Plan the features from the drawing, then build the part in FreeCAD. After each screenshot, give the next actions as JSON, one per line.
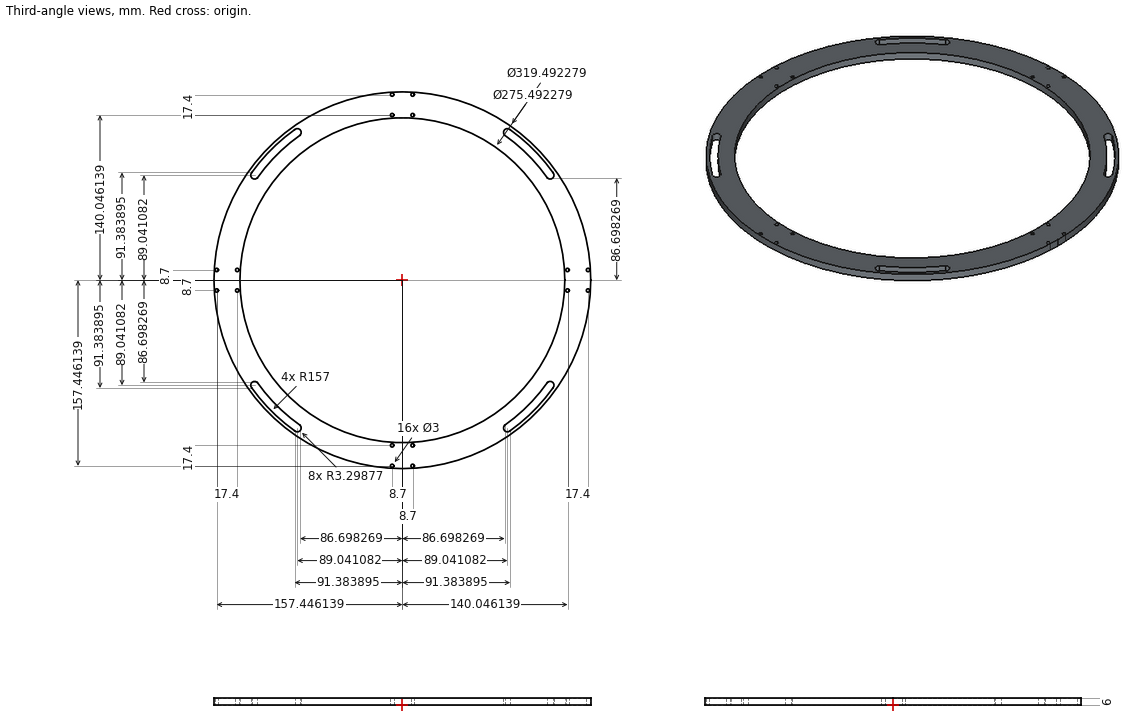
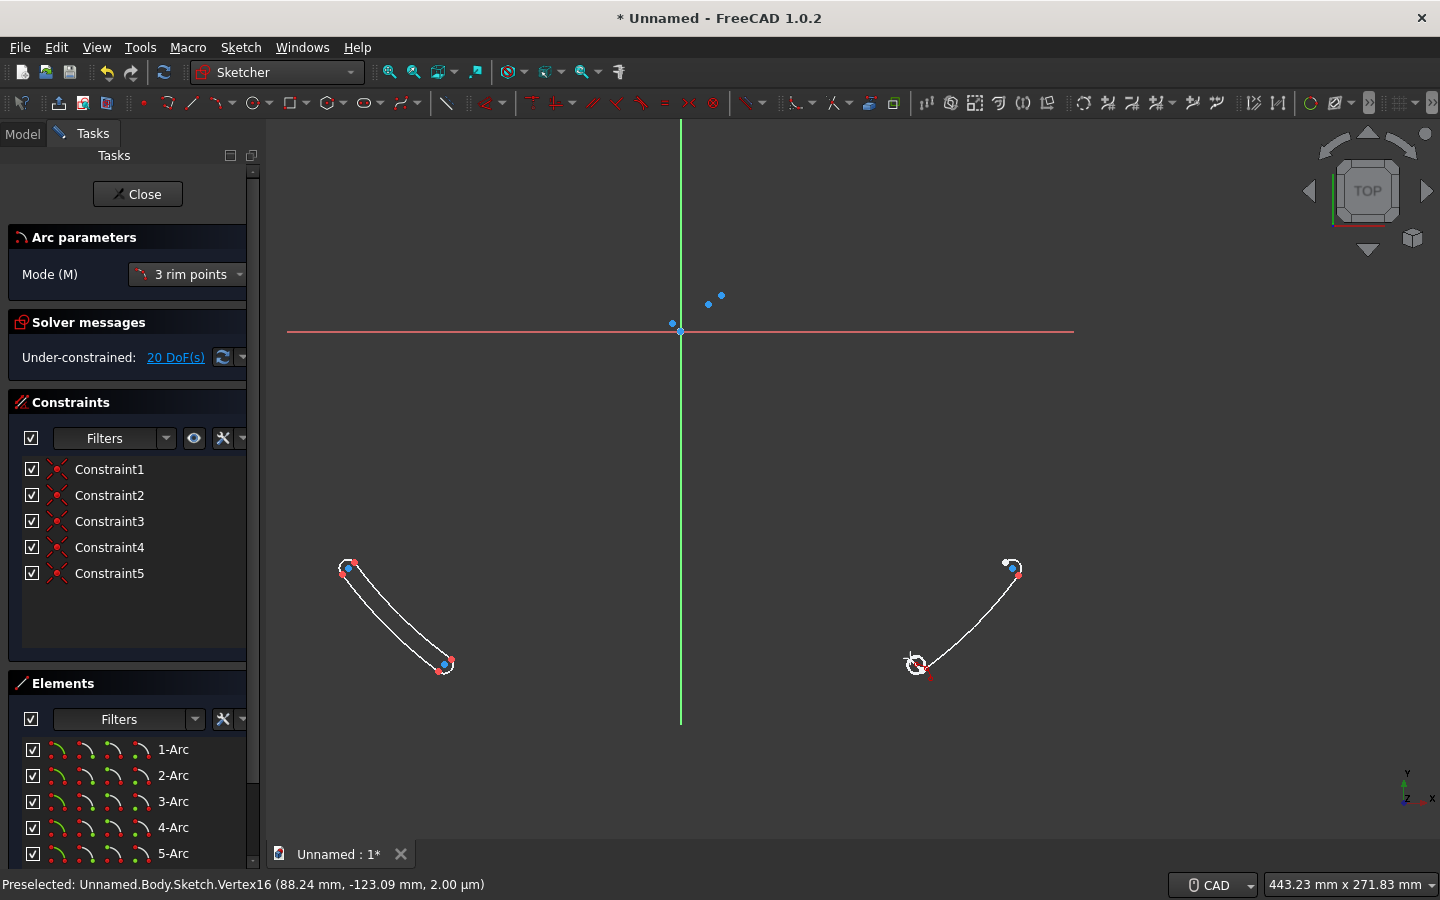
{"action": "scroll", "coordinate": [910, 670], "scroll_direction": "up", "scroll_amount": 3}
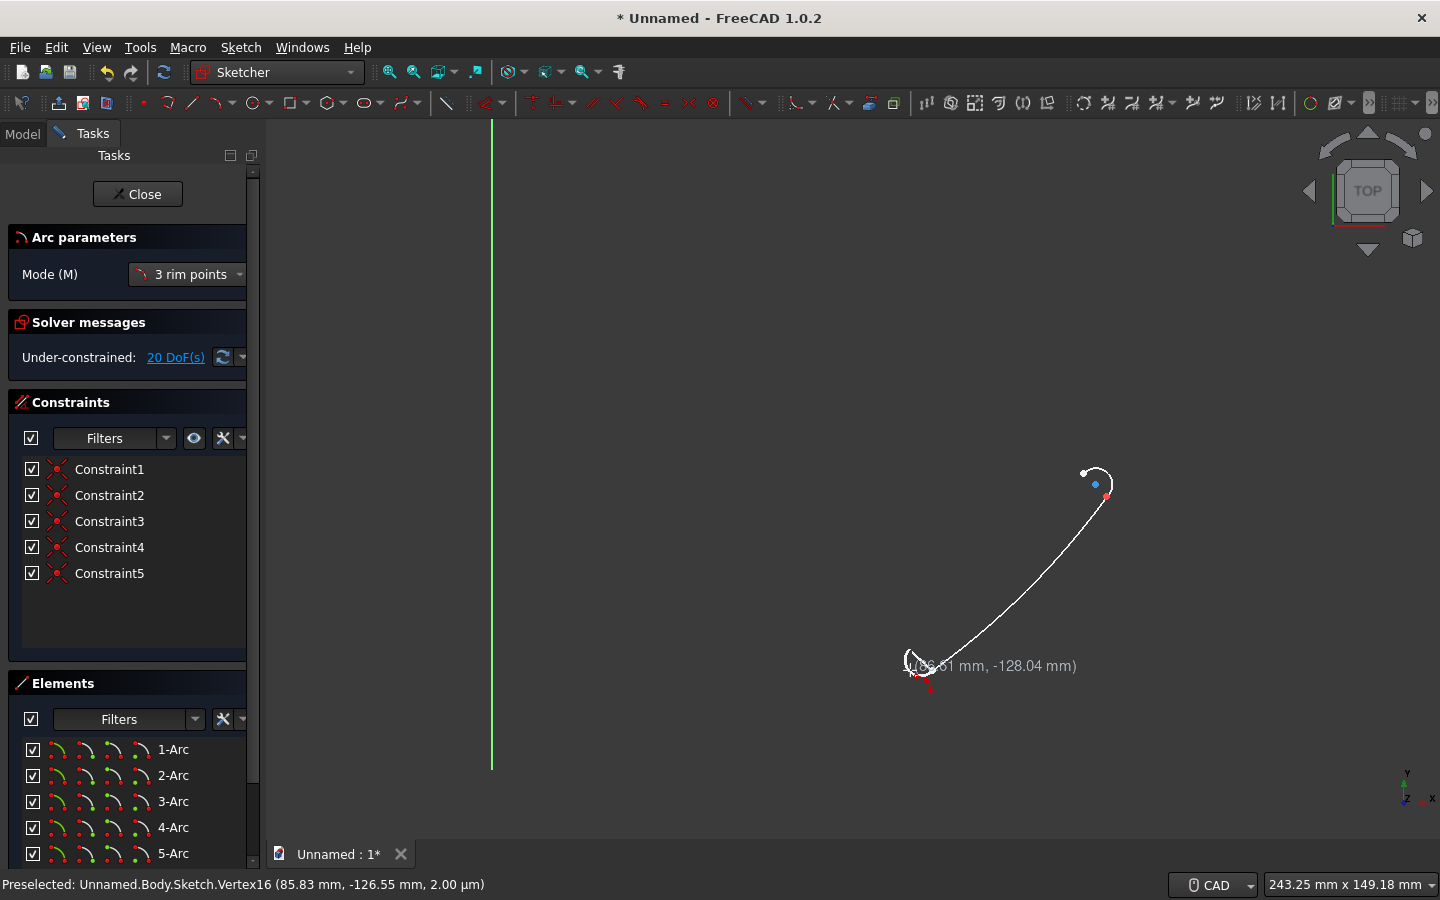
{"action": "left_click", "coordinate": [910, 669]}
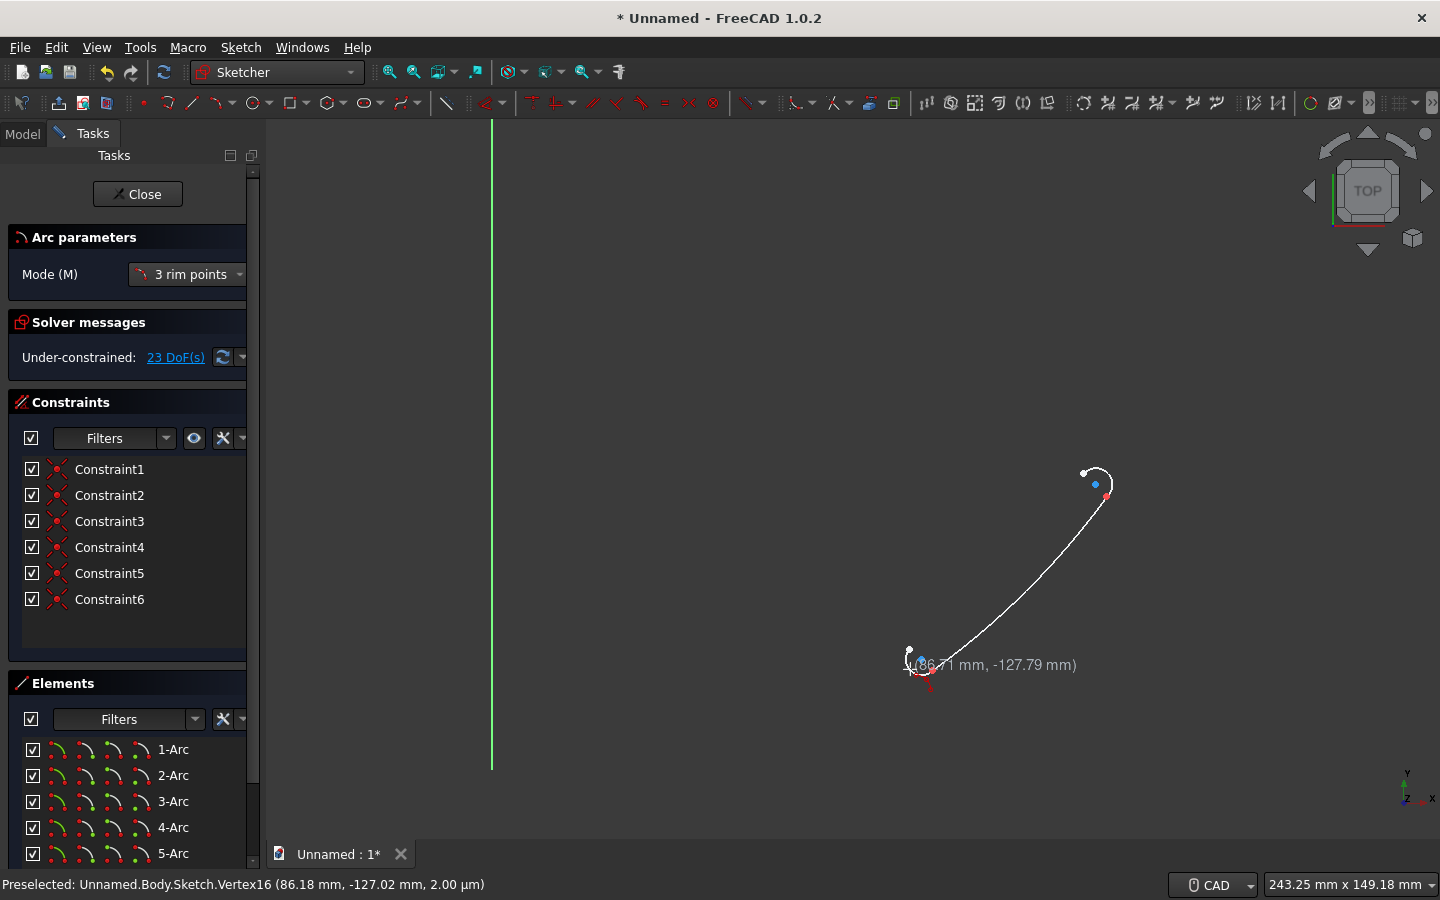
{"action": "left_click", "coordinate": [910, 649]}
{"action": "left_click", "coordinate": [1084, 474]}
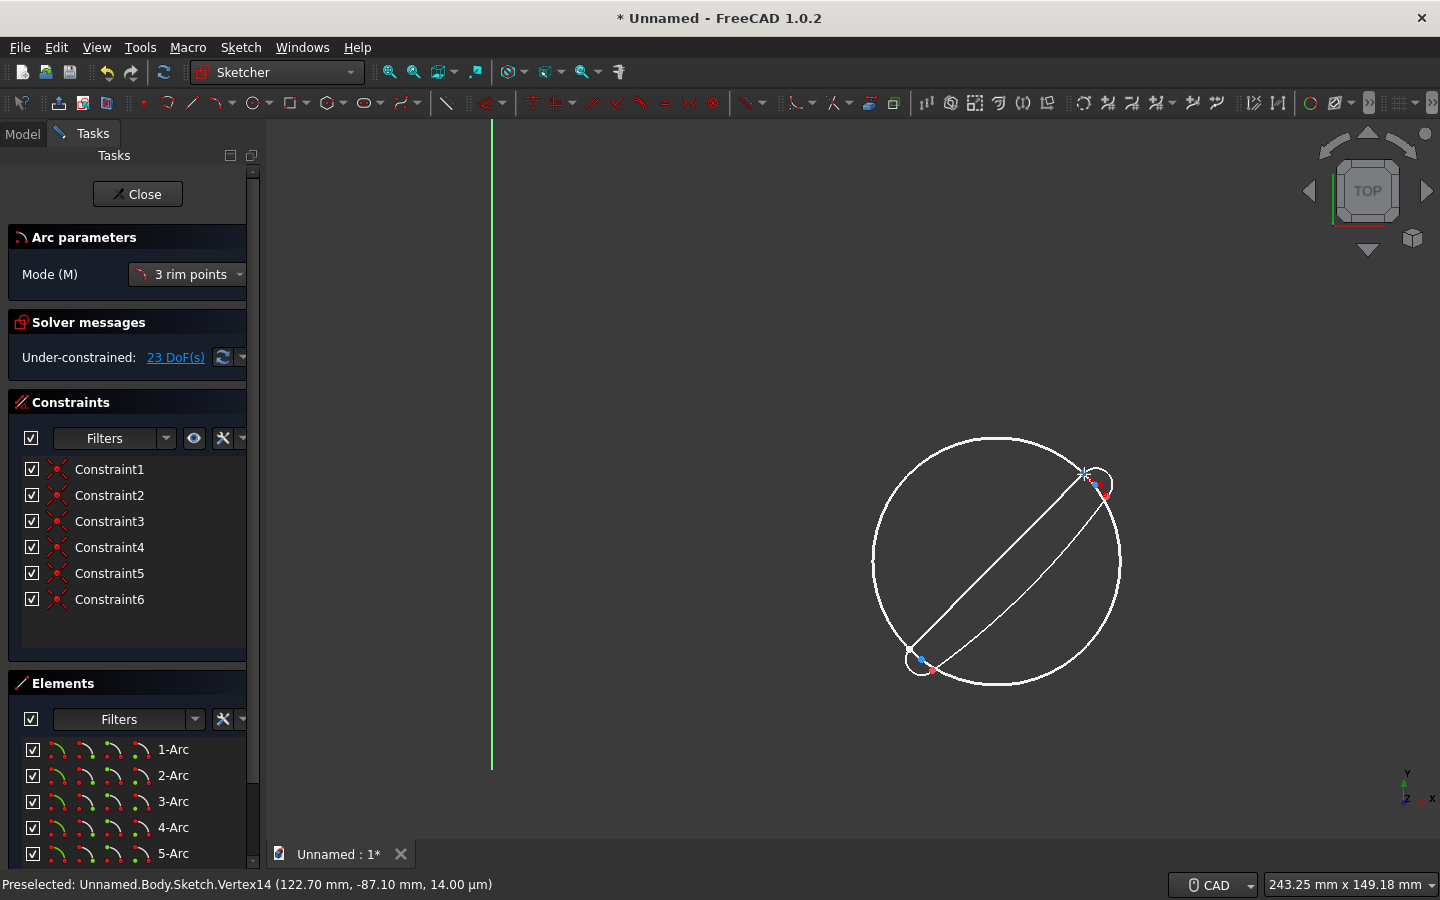
{"action": "scroll", "coordinate": [1005, 567], "scroll_direction": "up", "scroll_amount": 2}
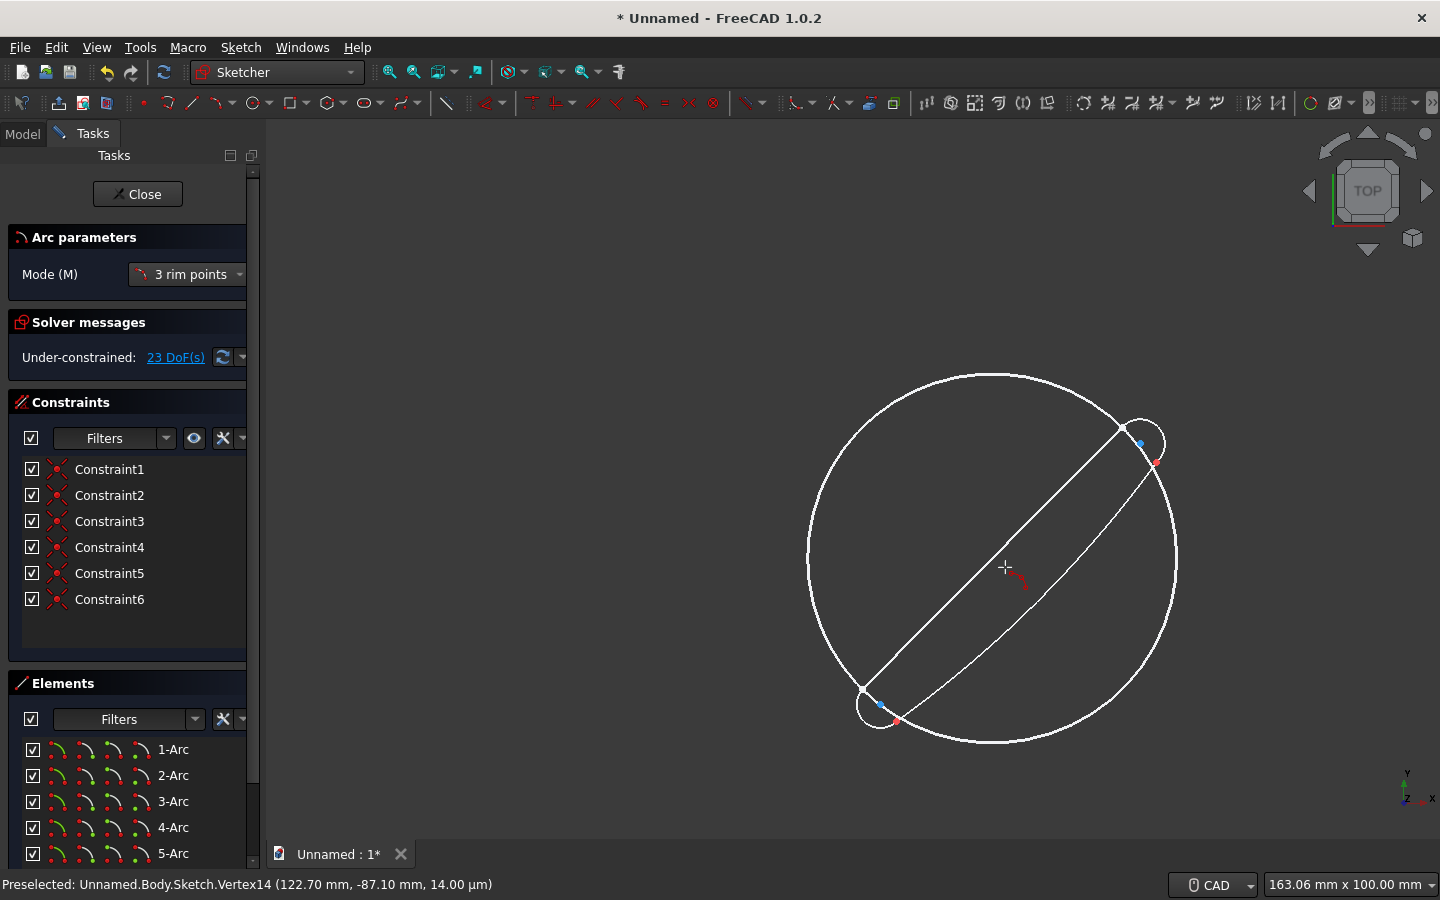
{"action": "left_click", "coordinate": [1005, 566]}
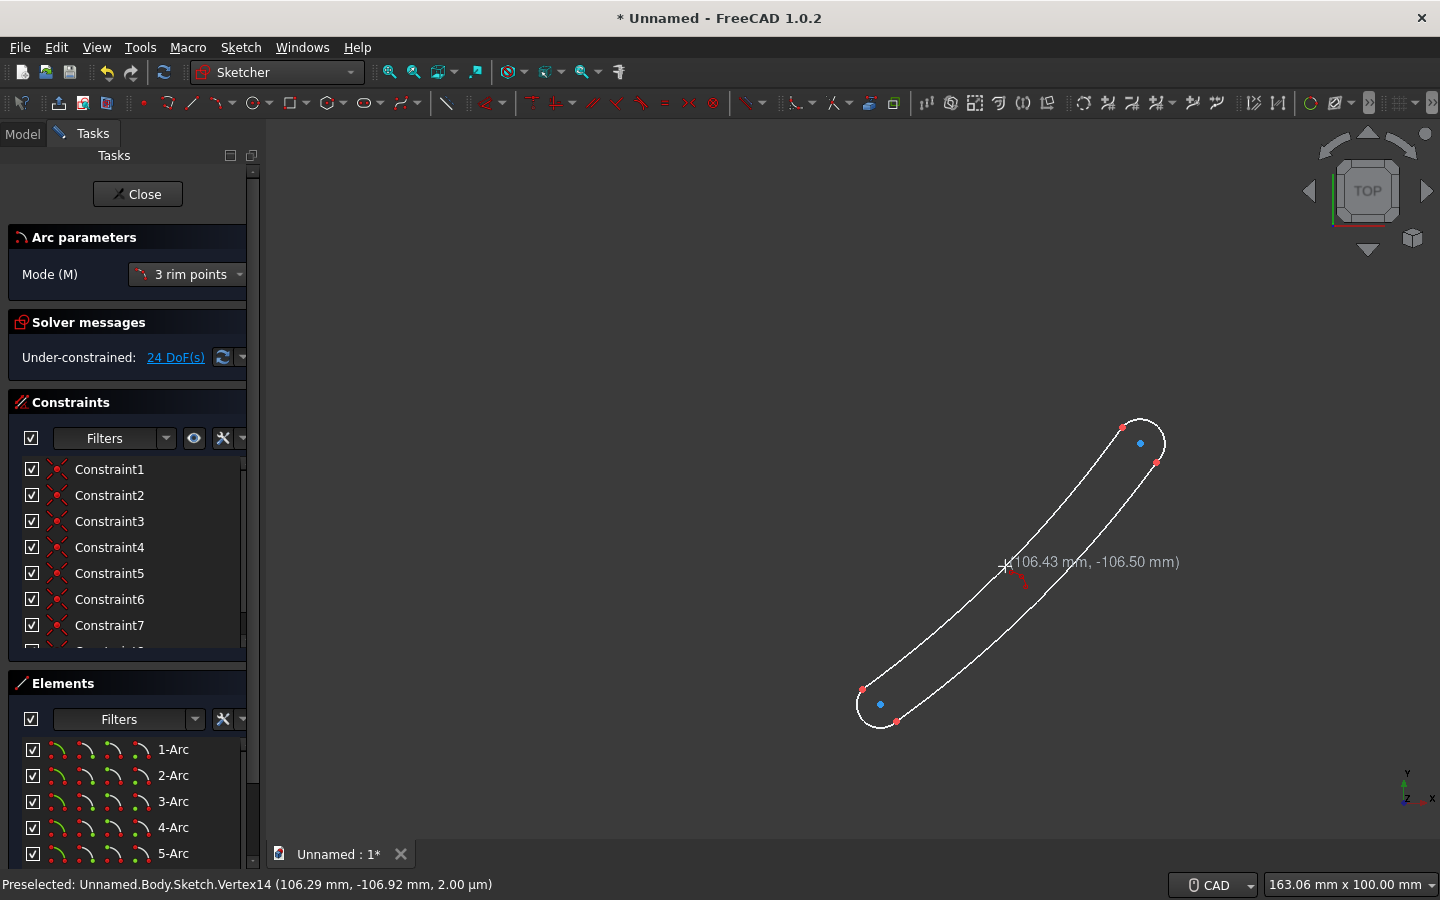
{"action": "scroll", "coordinate": [923, 651], "scroll_direction": "down", "scroll_amount": 8}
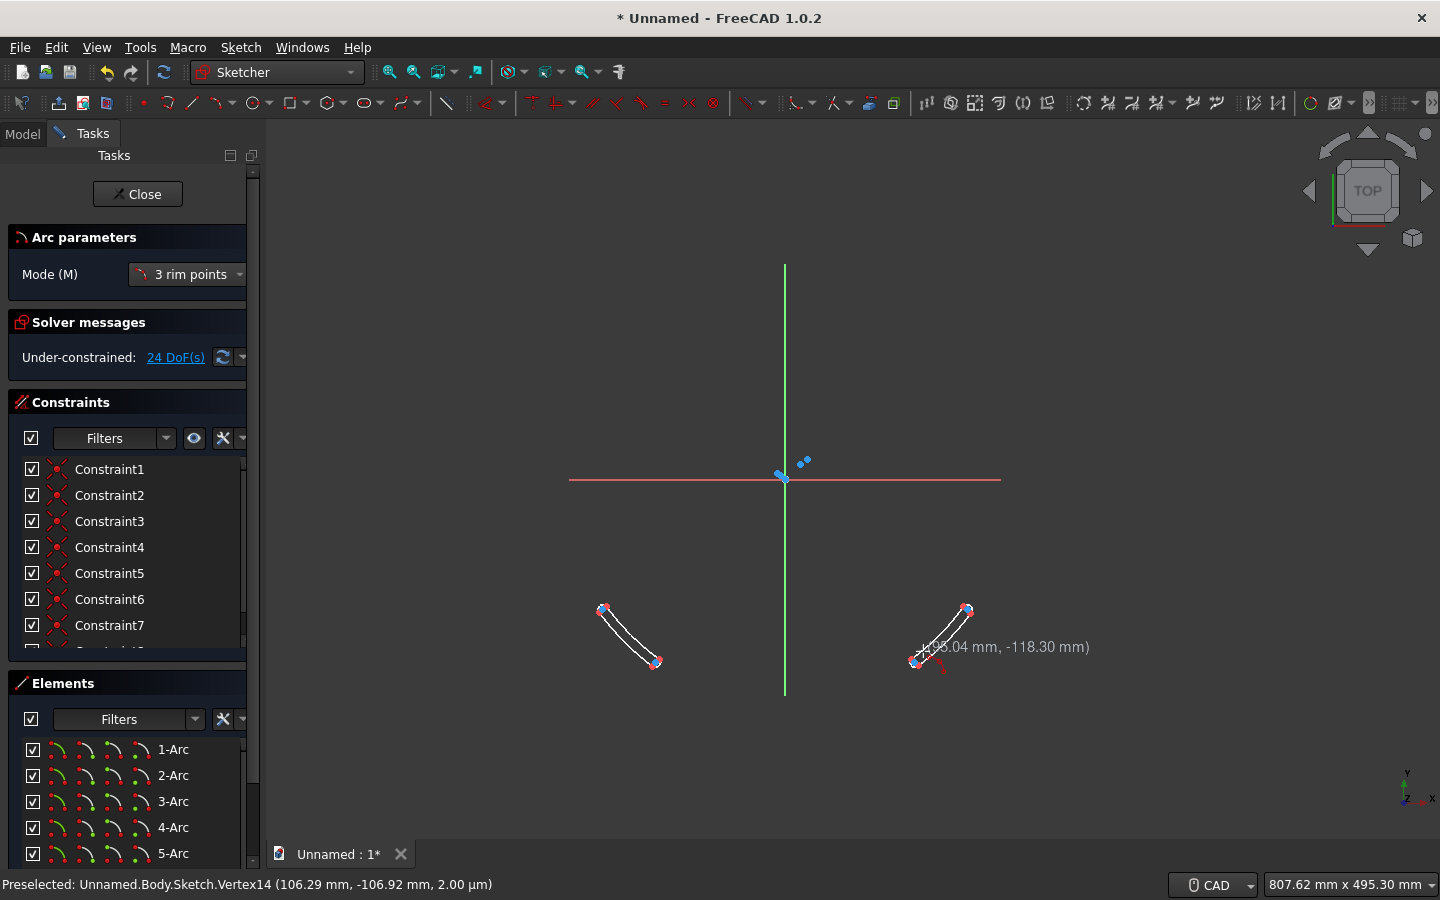
{"action": "left_click", "coordinate": [606, 354]}
{"action": "left_click", "coordinate": [600, 347]}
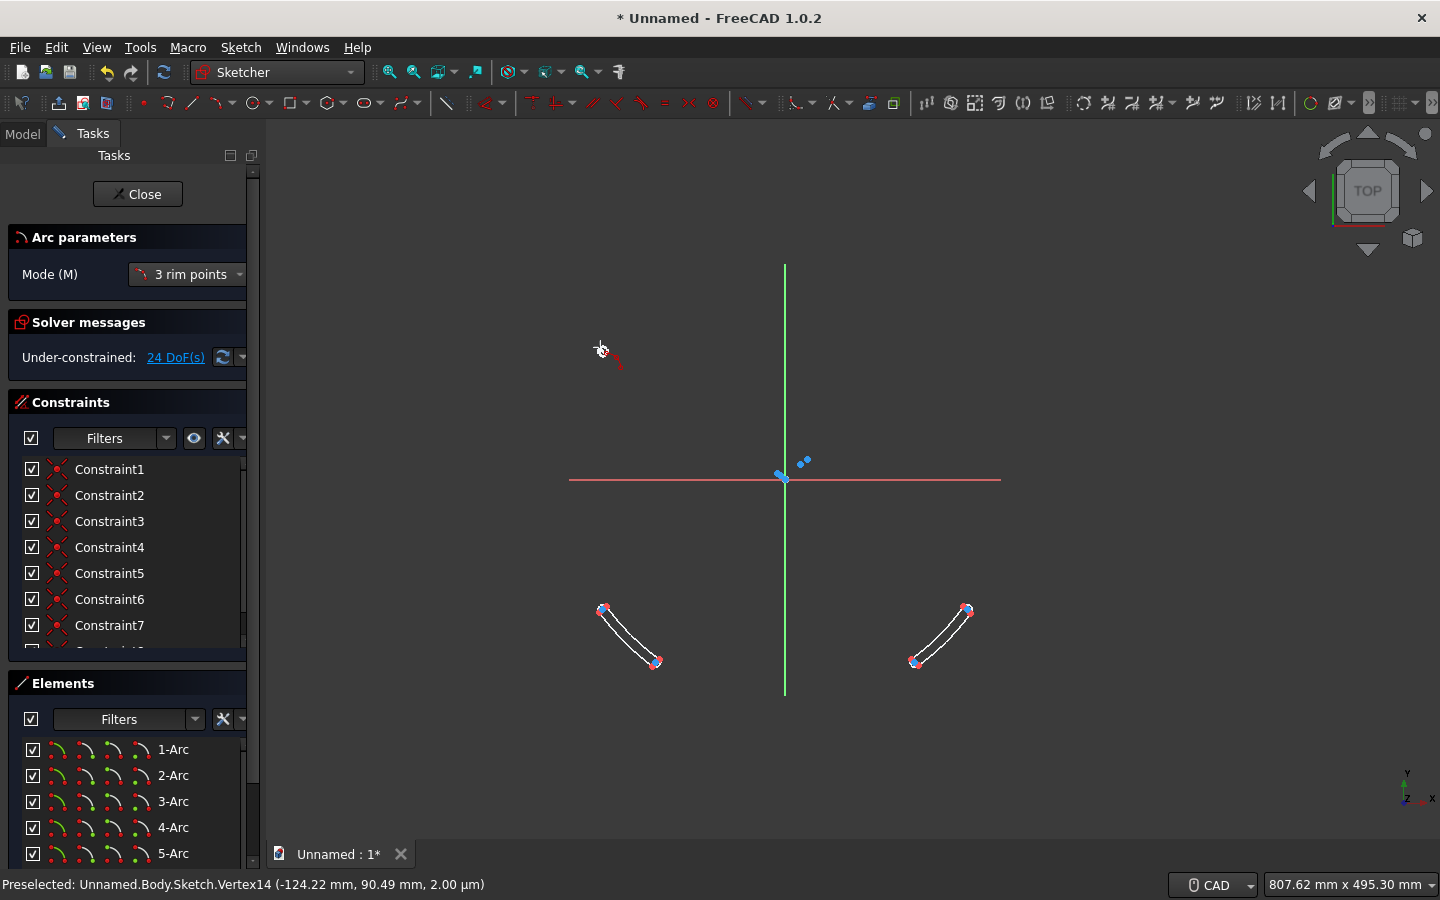
{"action": "scroll", "coordinate": [600, 354], "scroll_direction": "up", "scroll_amount": 6}